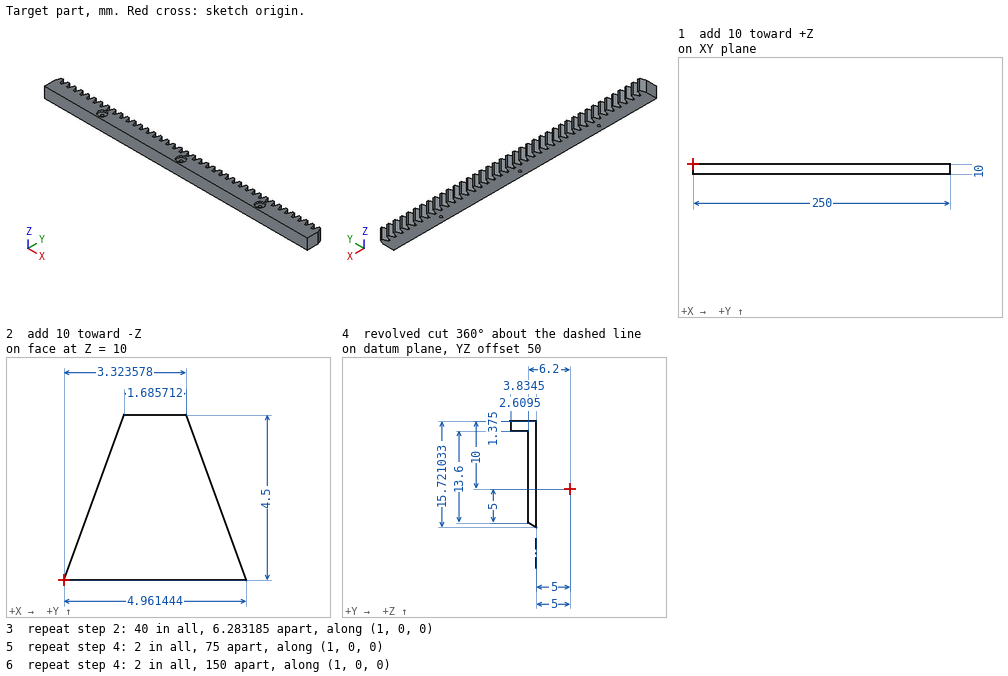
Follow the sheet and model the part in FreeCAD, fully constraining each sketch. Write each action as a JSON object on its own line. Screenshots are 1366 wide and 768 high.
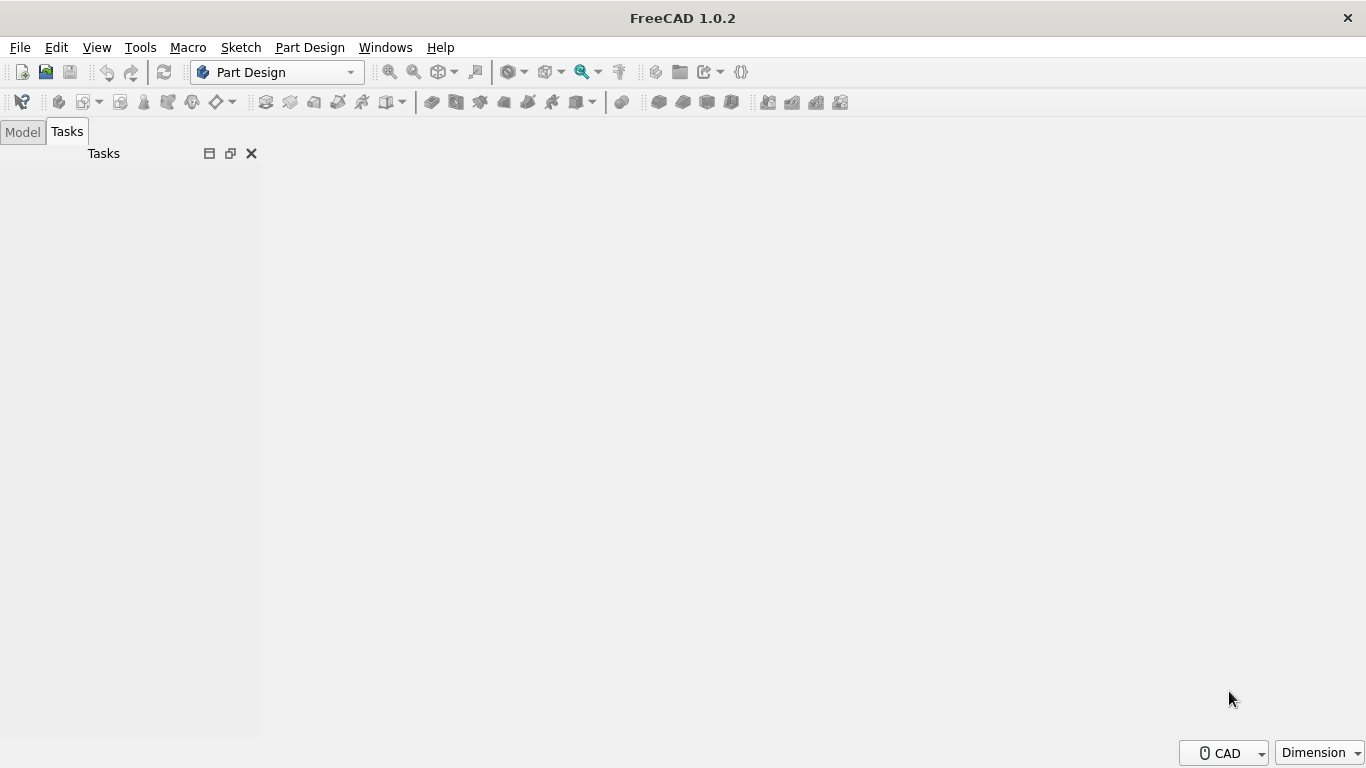
{"action": "left_click", "coordinate": [22, 72]}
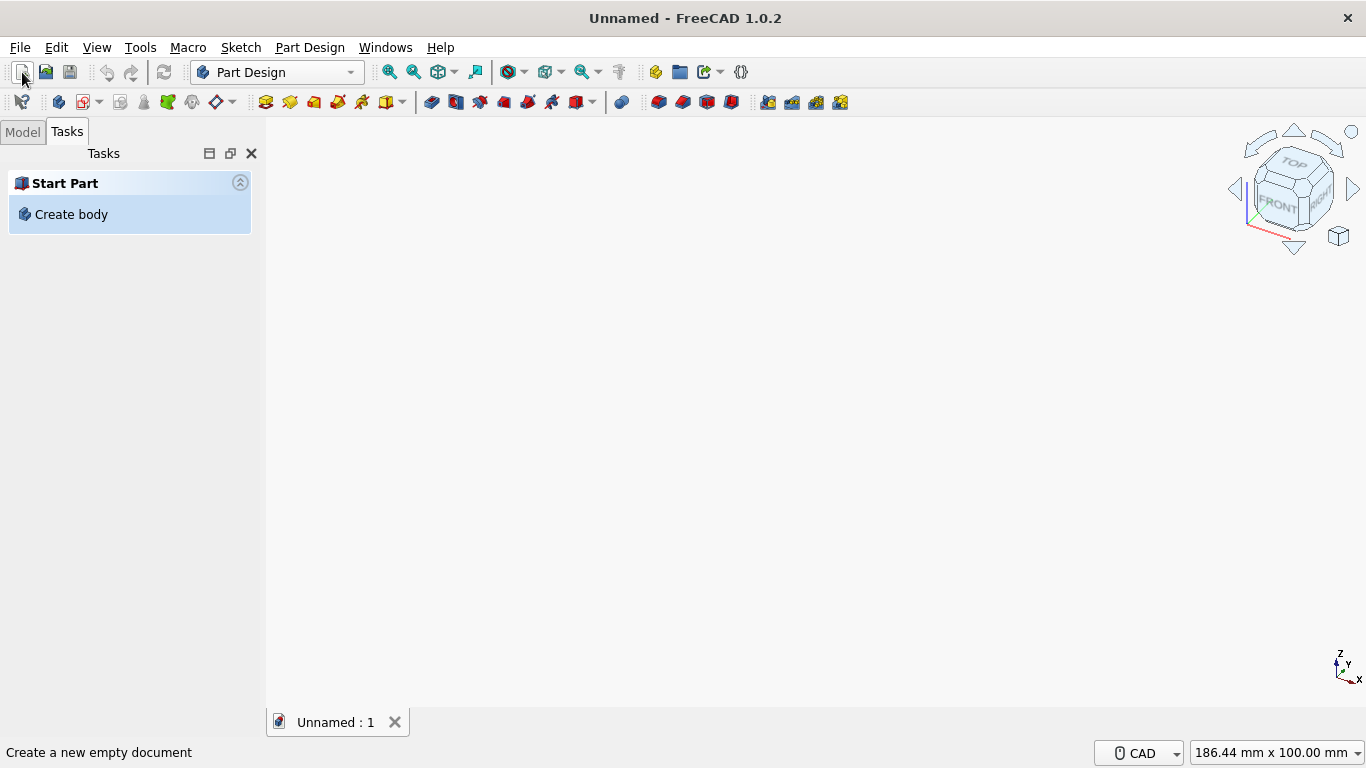
{"action": "left_click", "coordinate": [84, 102]}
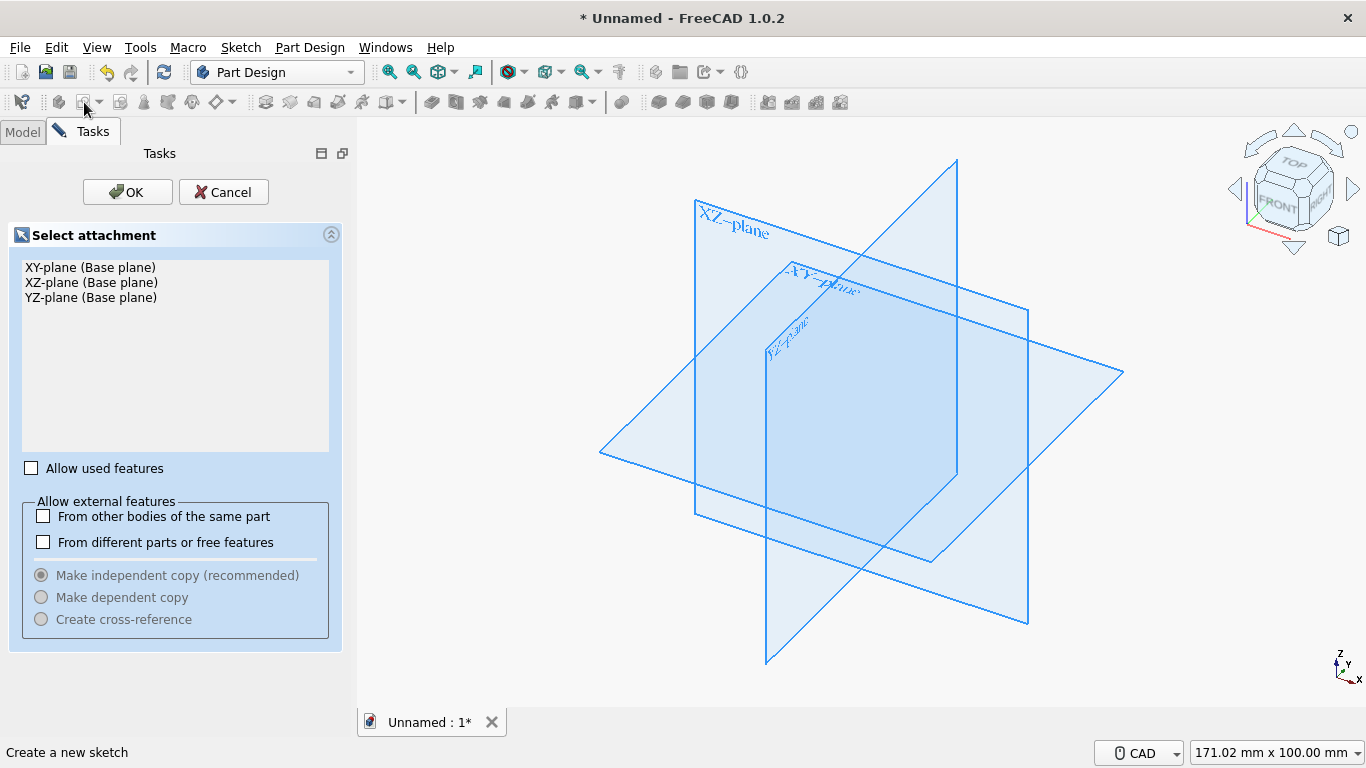
{"action": "left_click", "coordinate": [82, 268]}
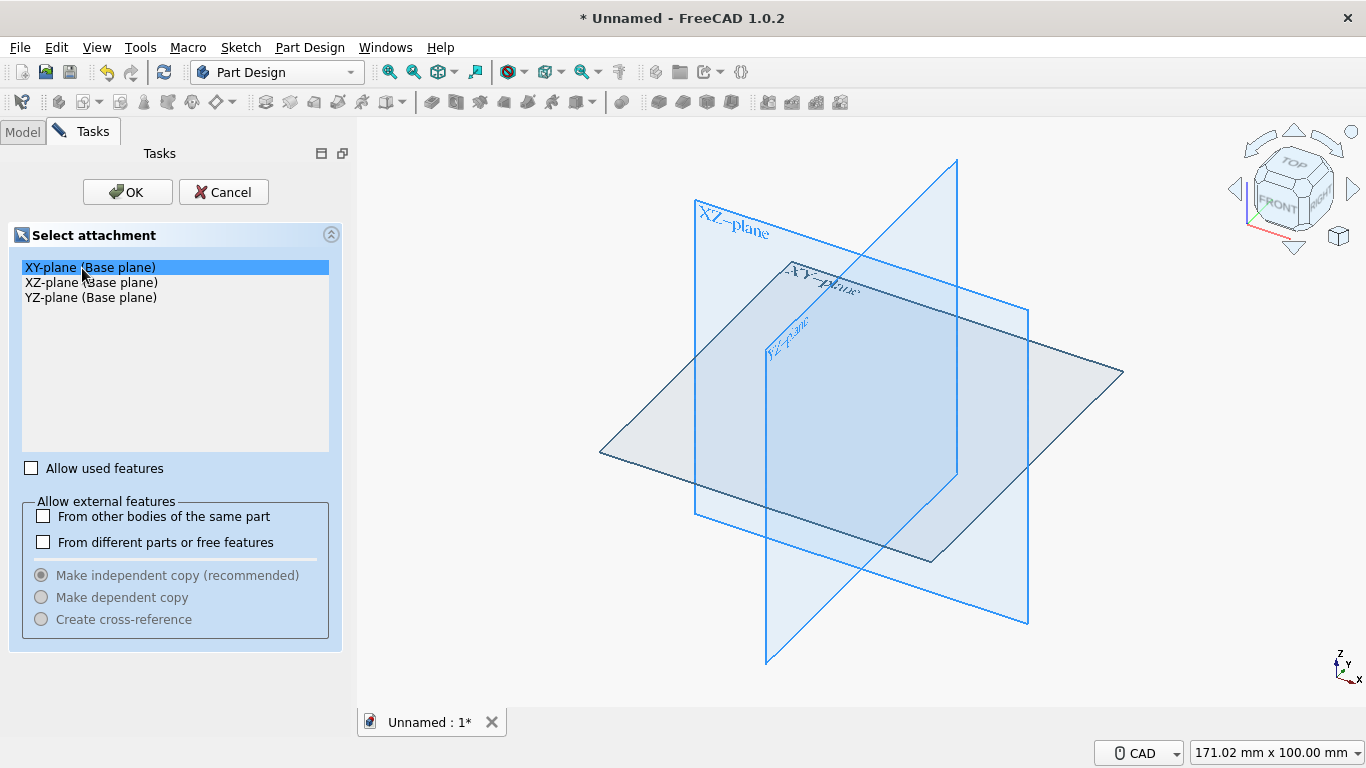
{"action": "left_click", "coordinate": [128, 192]}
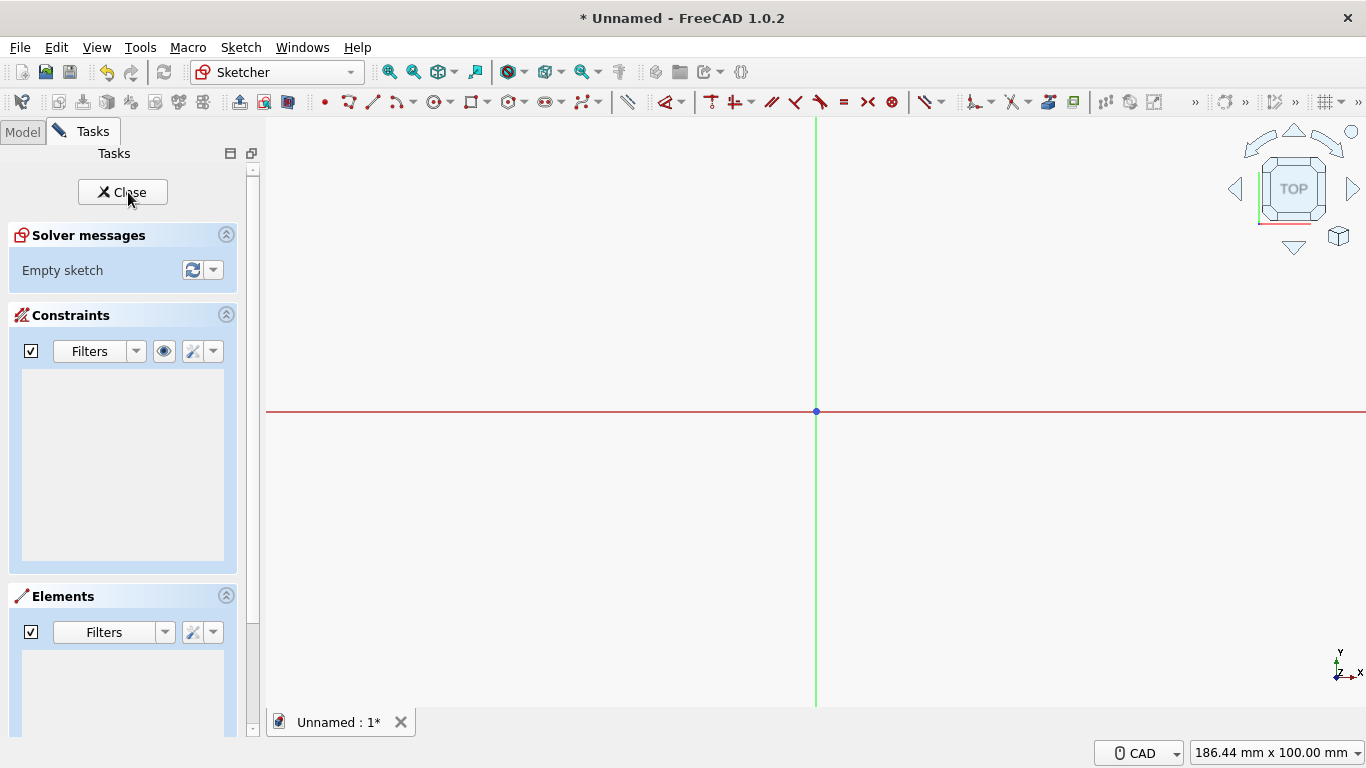
{"action": "scroll", "coordinate": [294, 395], "scroll_direction": "down", "scroll_amount": 5}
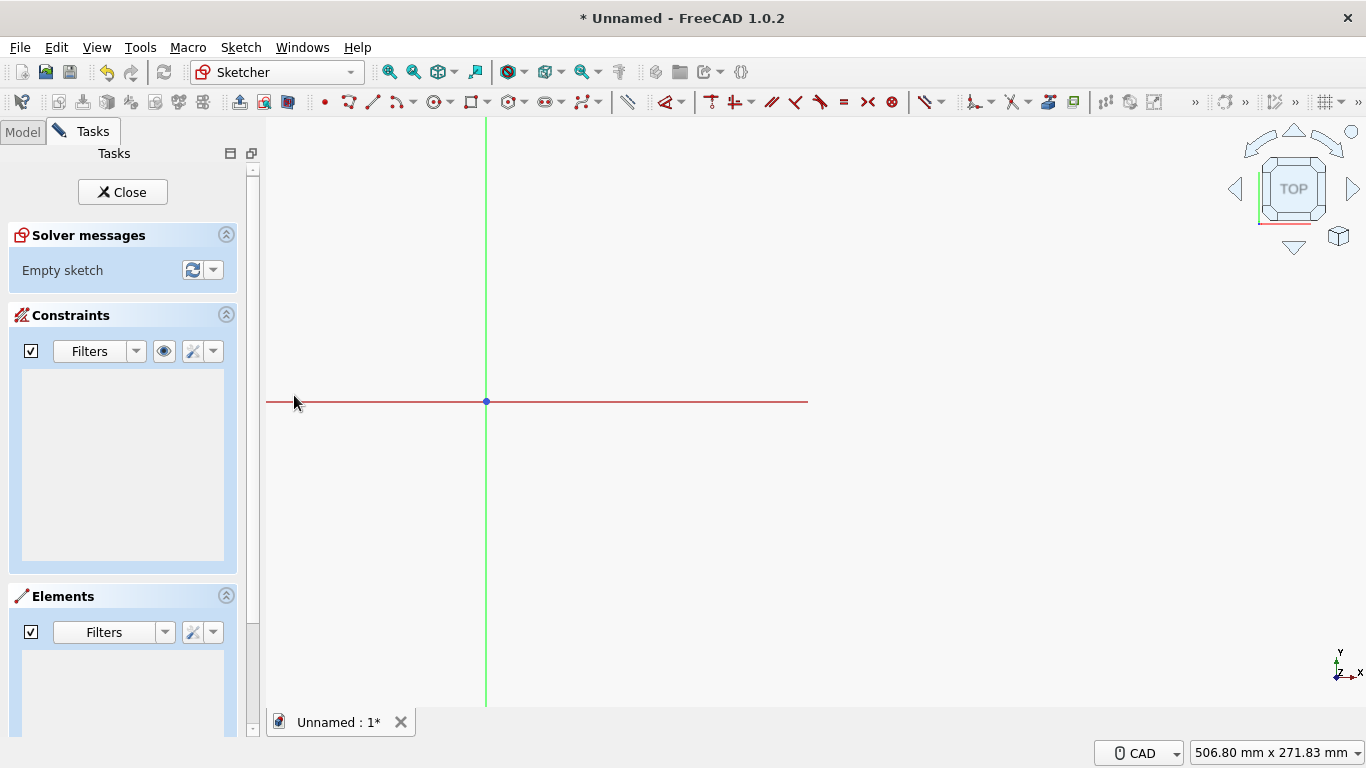
{"action": "left_click", "coordinate": [472, 102]}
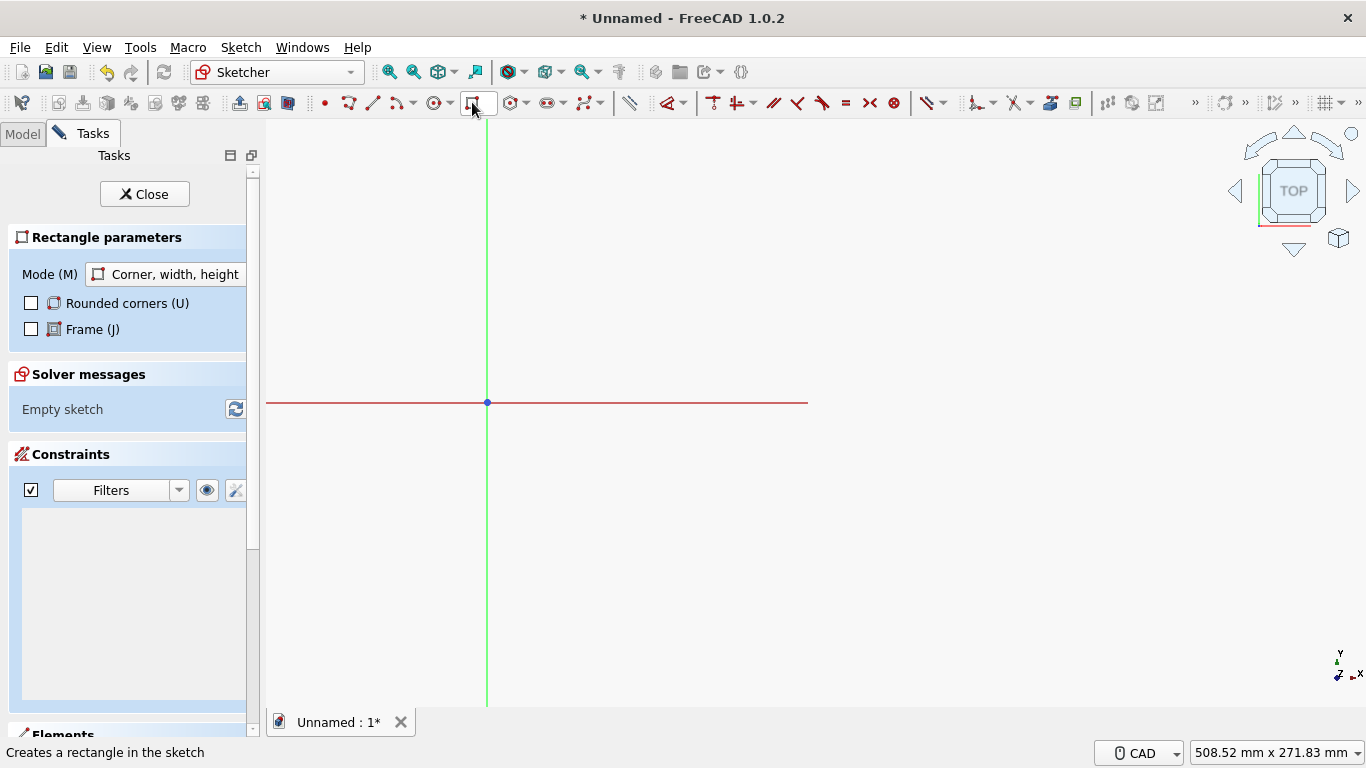
{"action": "left_click", "coordinate": [487, 403]}
{"action": "mouse_move", "coordinate": [1028, 424]}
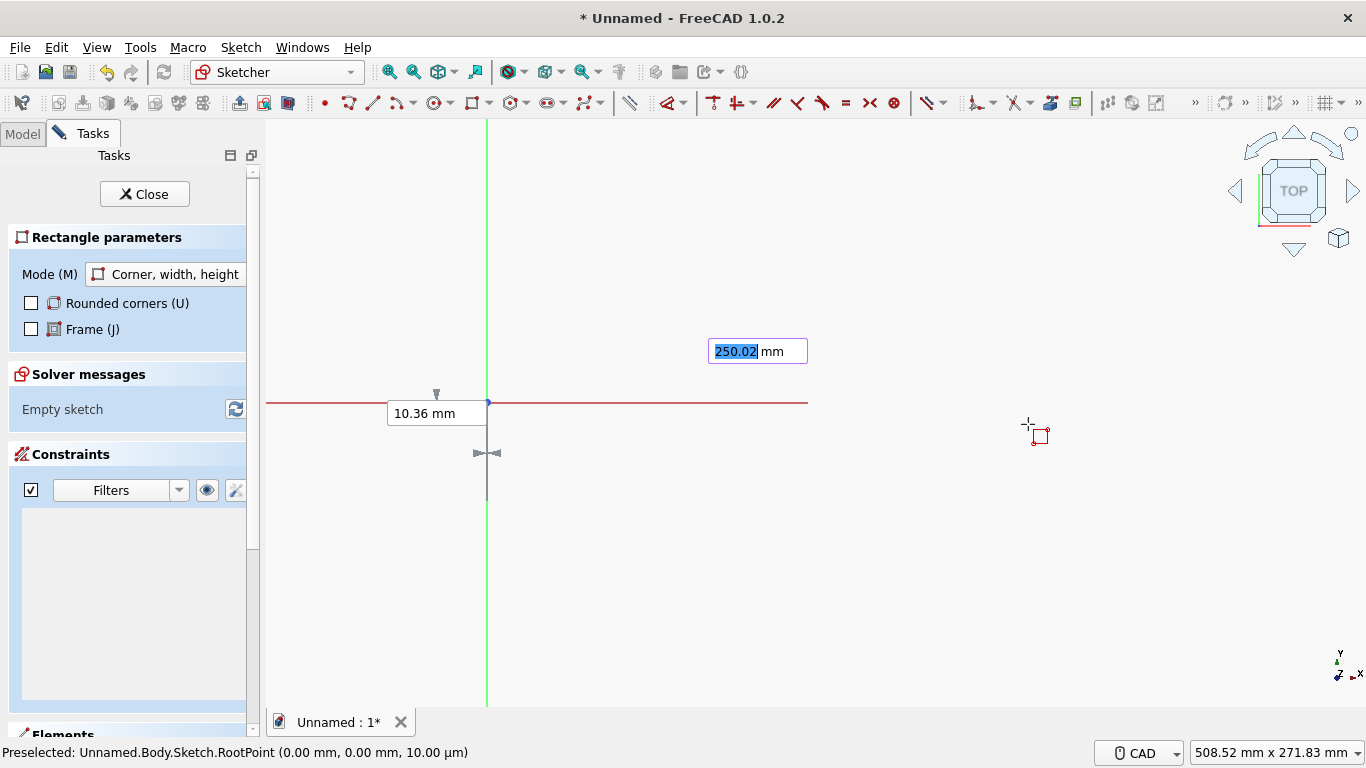
{"action": "type", "text": "250"}
{"action": "key", "text": "Tab"}
{"action": "type", "text": "10"}
{"action": "key", "text": "Return"}
{"action": "key", "text": "Escape"}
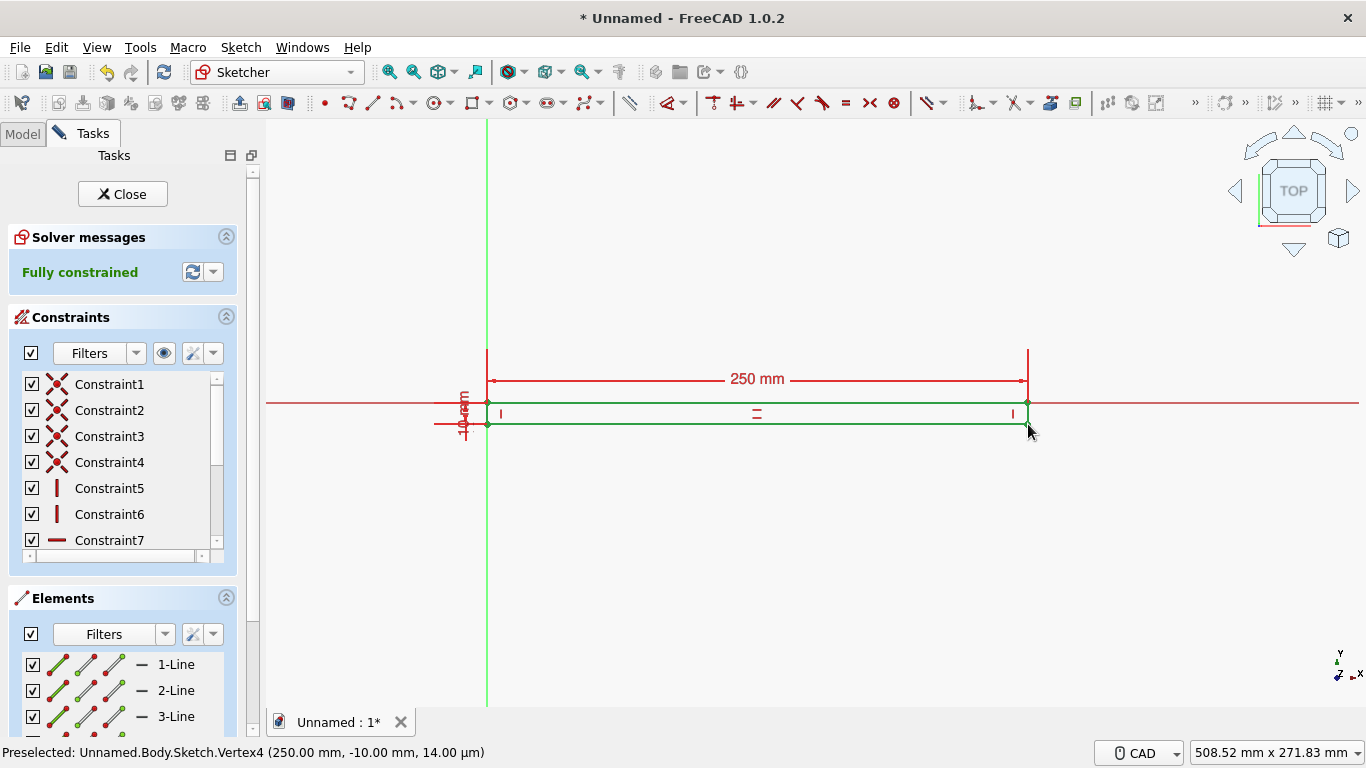
{"action": "left_click", "coordinate": [123, 194]}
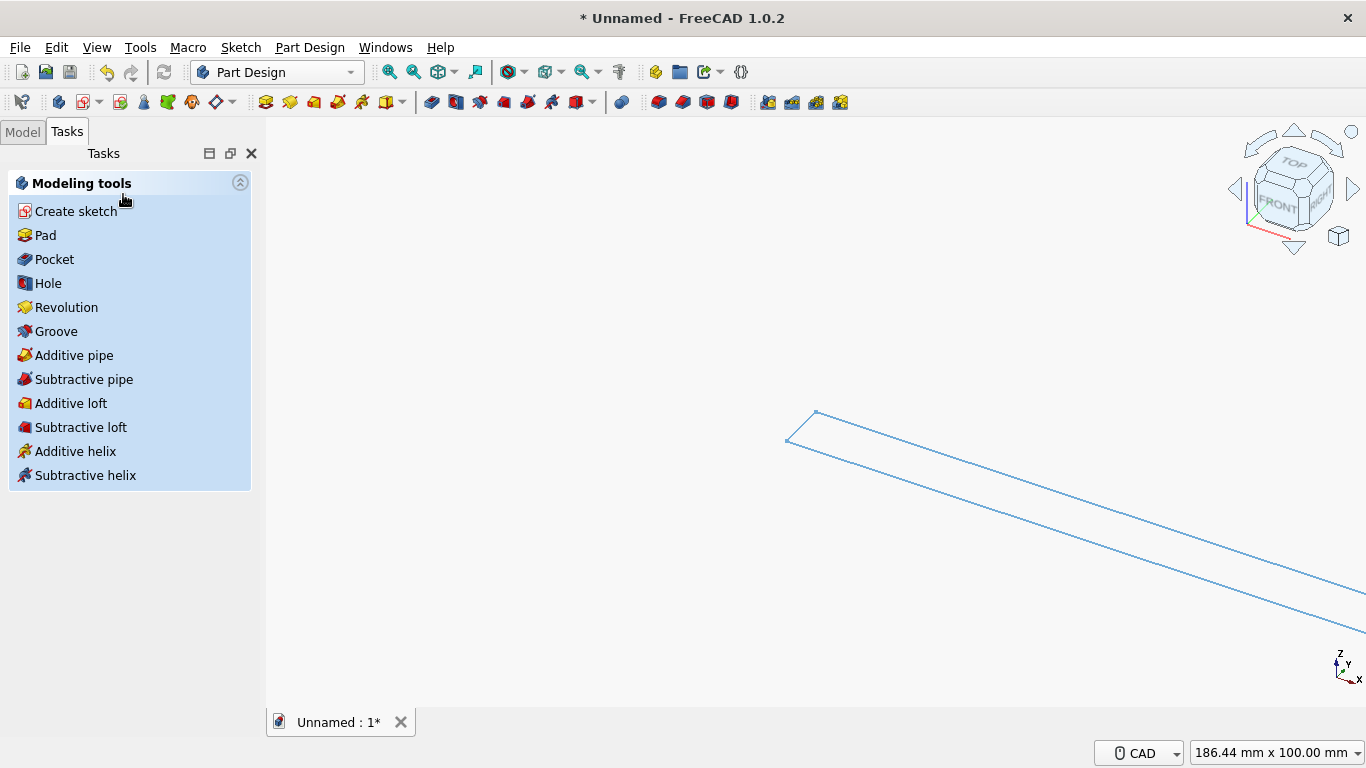
{"action": "left_click", "coordinate": [266, 102]}